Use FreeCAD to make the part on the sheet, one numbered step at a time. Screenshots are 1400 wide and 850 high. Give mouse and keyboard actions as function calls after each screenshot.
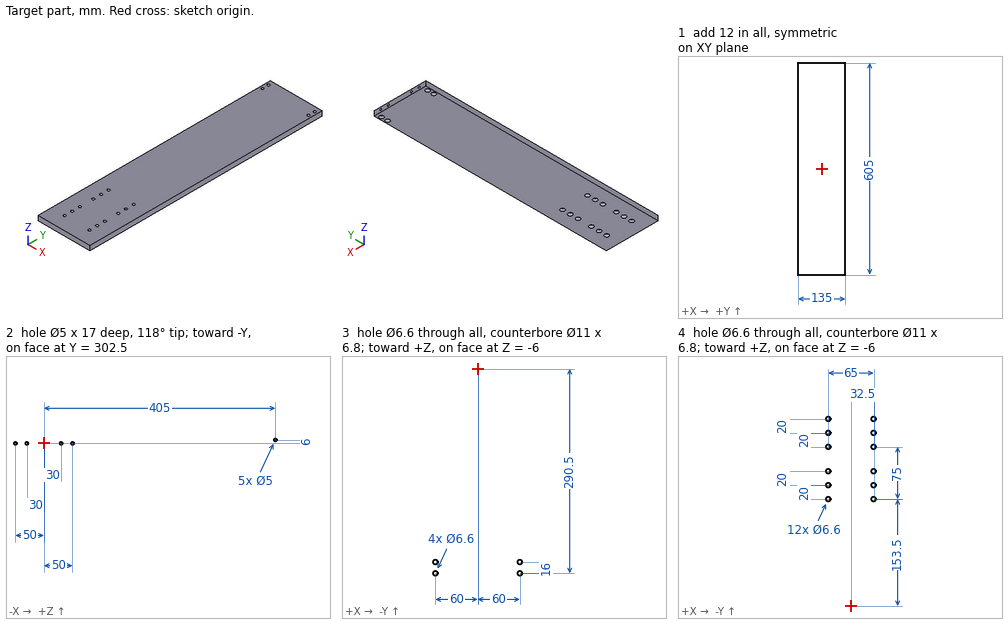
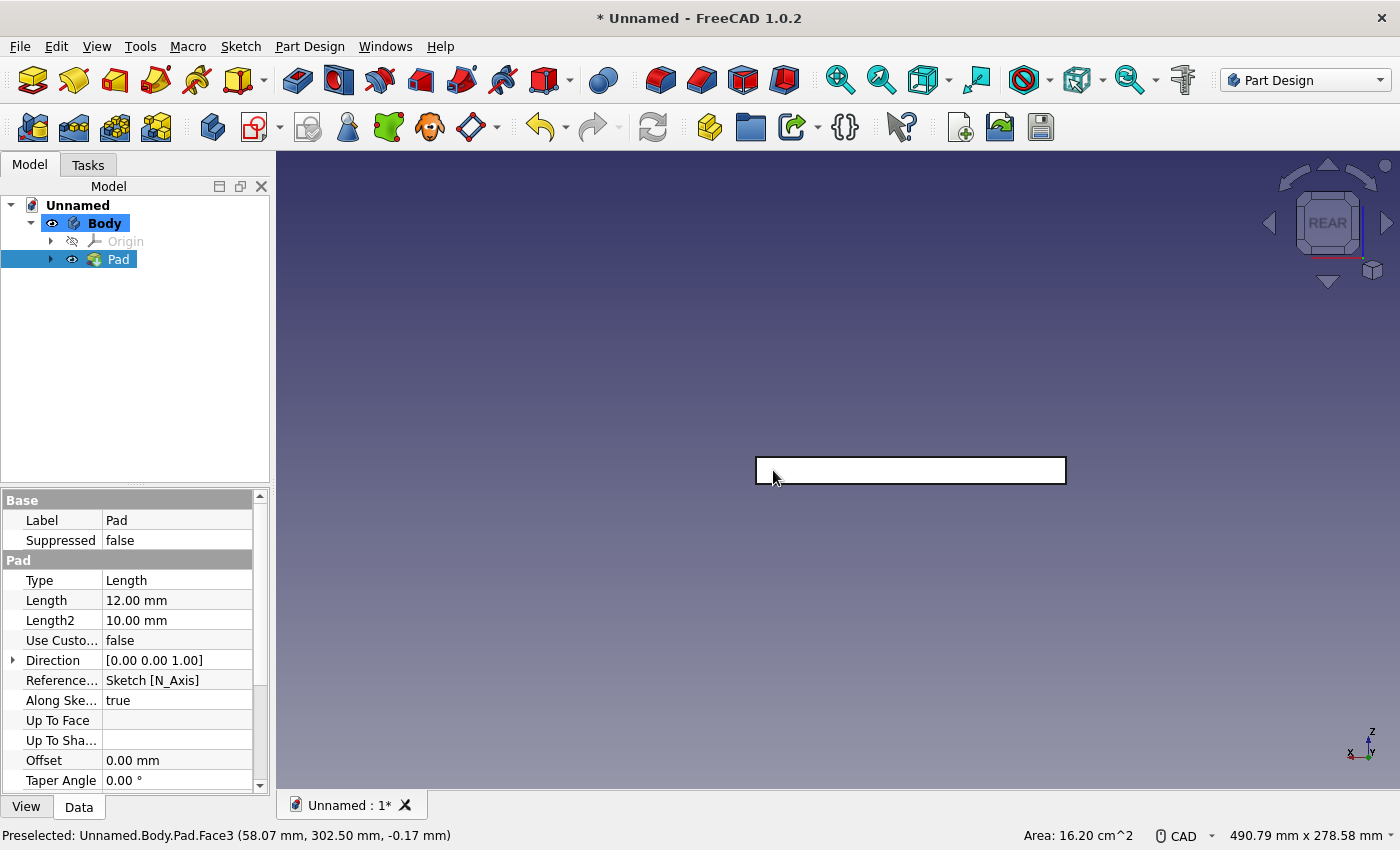
click(254, 128)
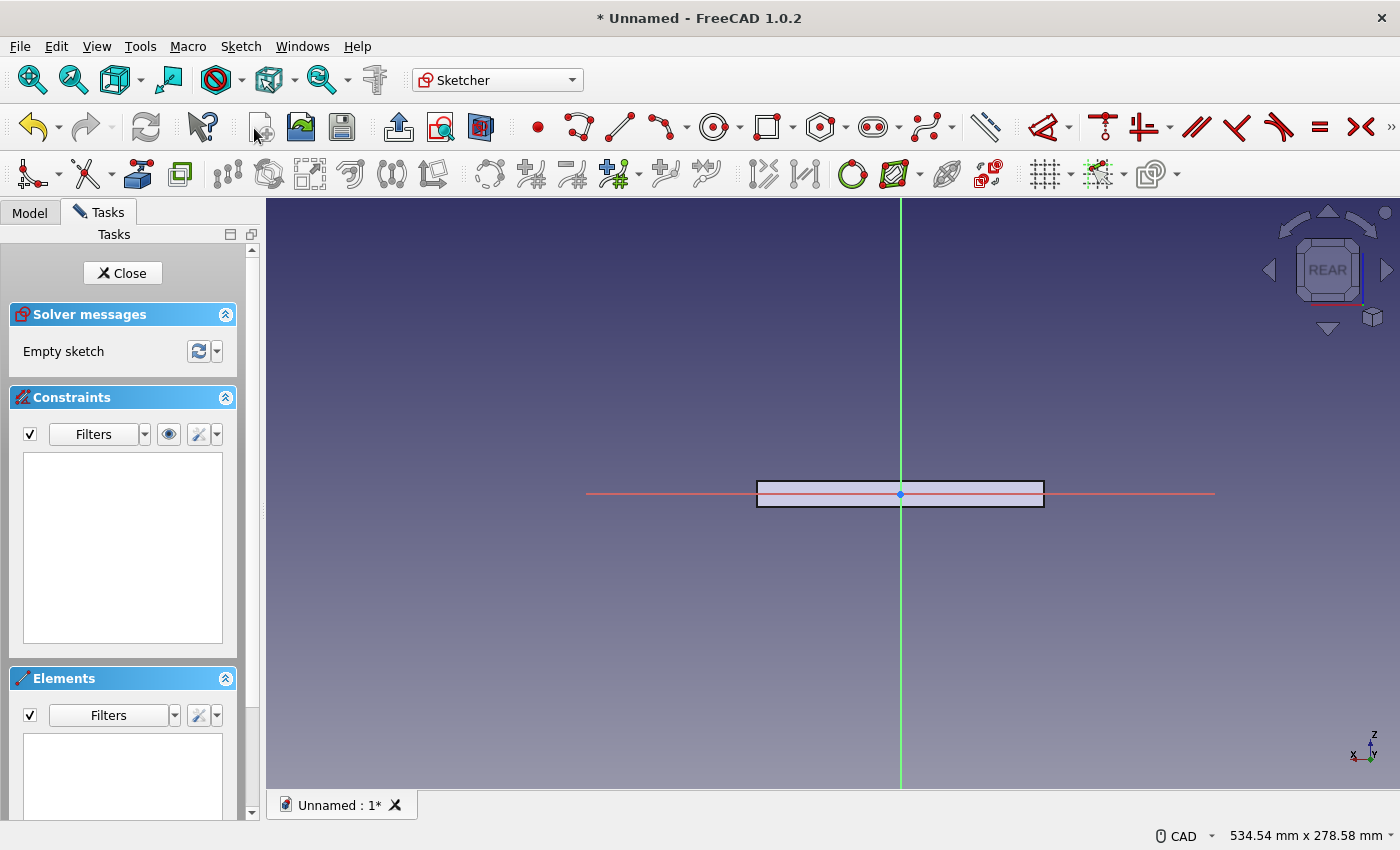
scroll(294, 501, down, 3)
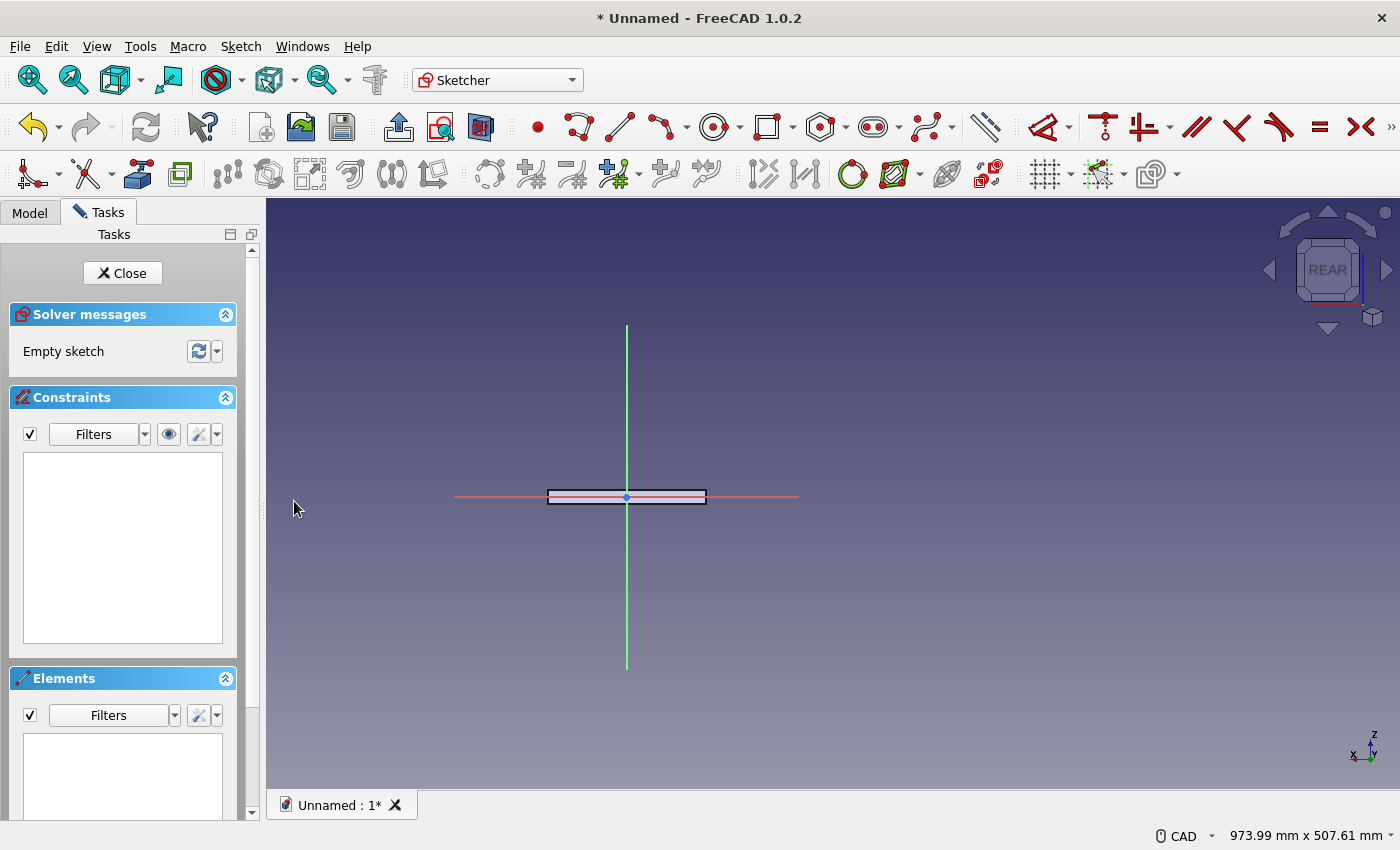
key(g)
key(c)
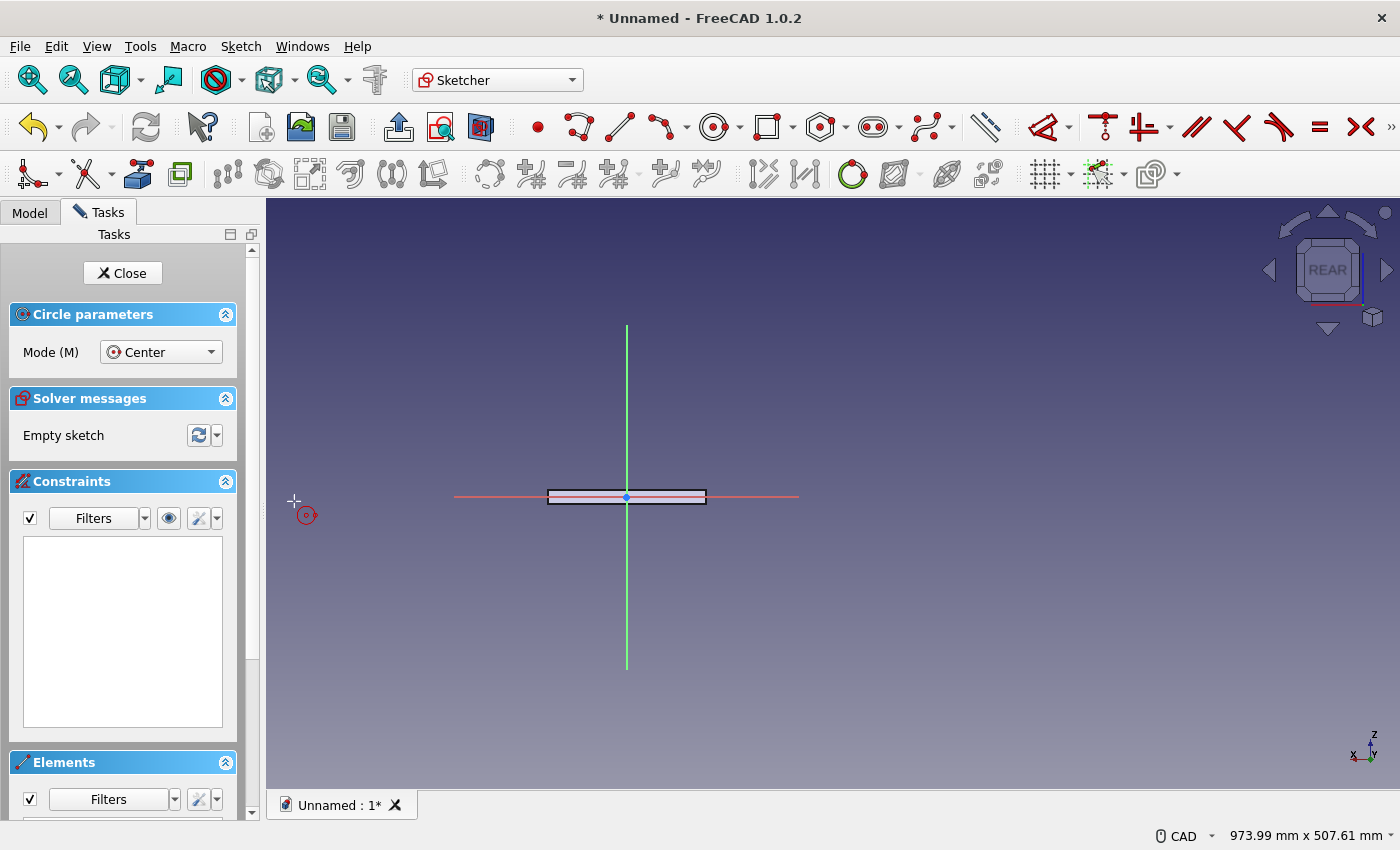
scroll(569, 497, up, 11)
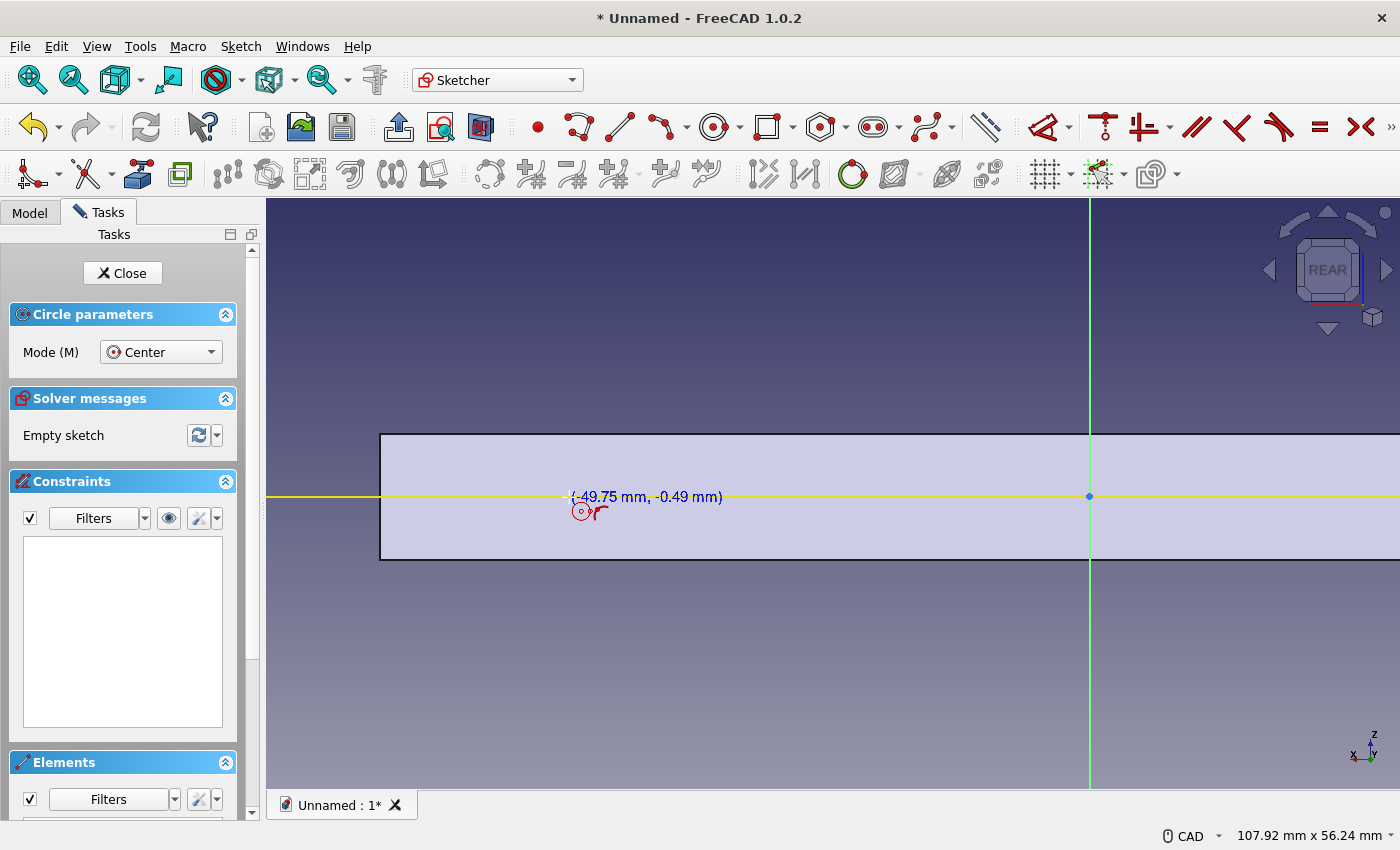
scroll(422, 498, down, 10)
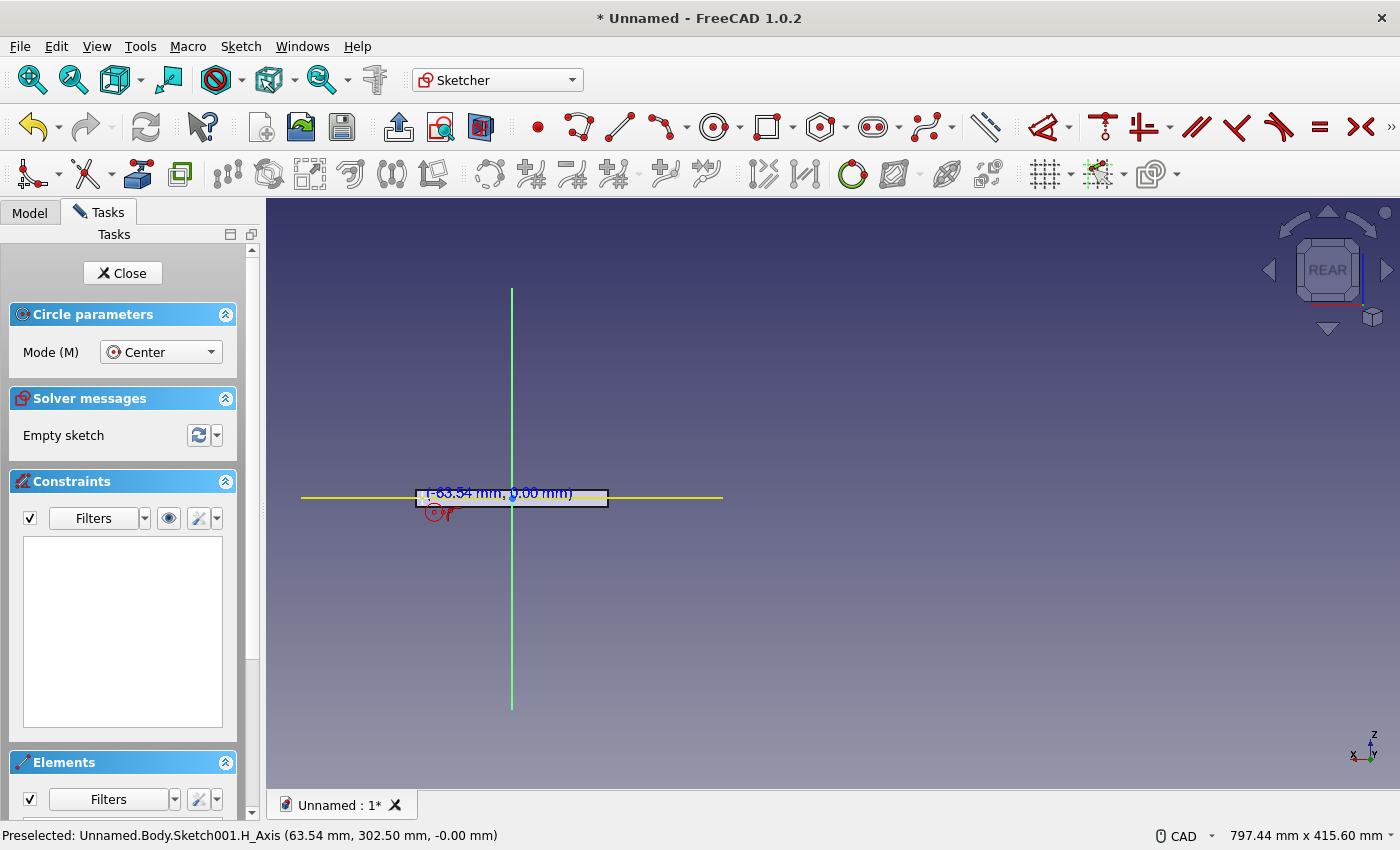
click(441, 498)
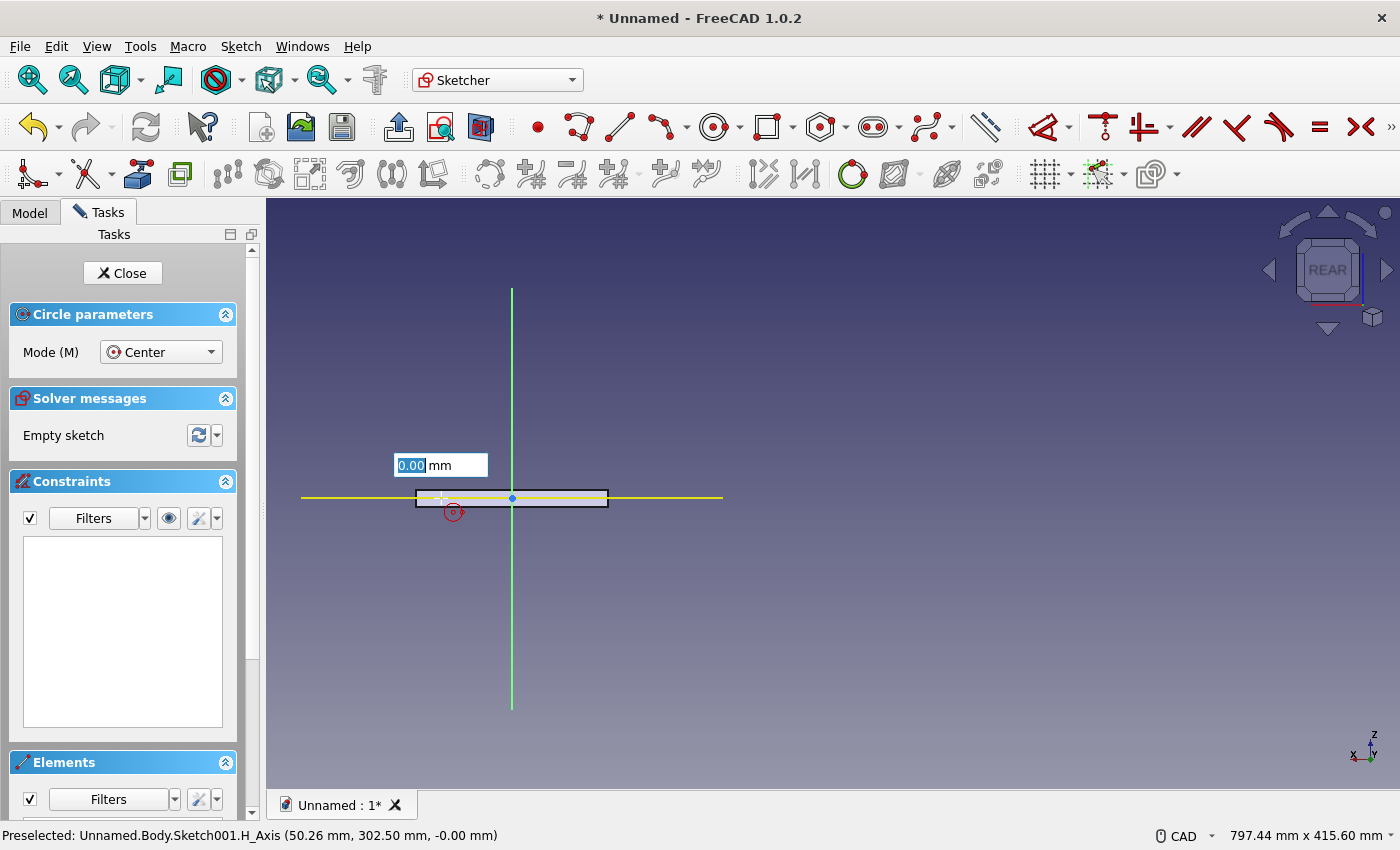
scroll(440, 502, up, 8)
move(440, 498)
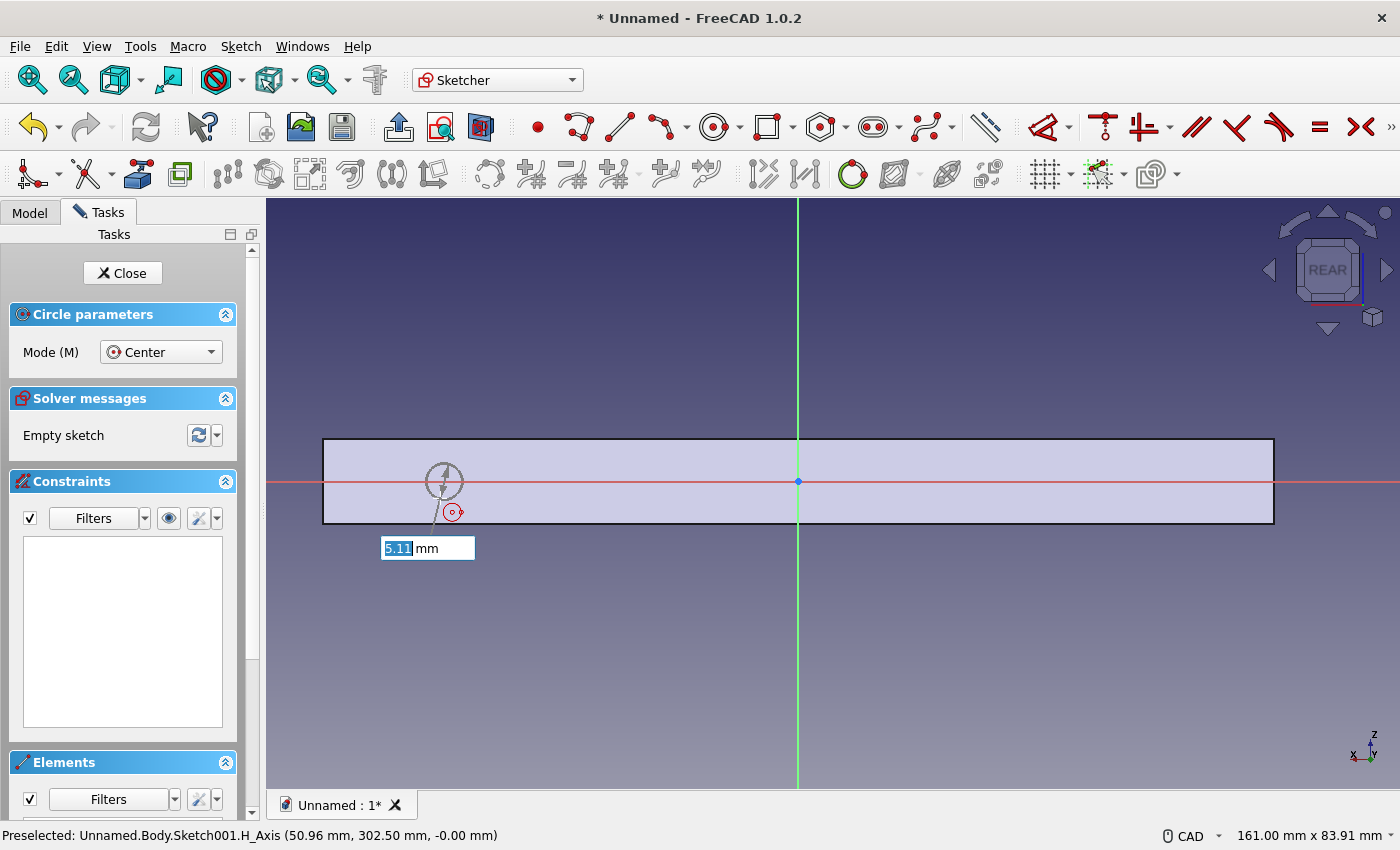
text(5)
key(Return)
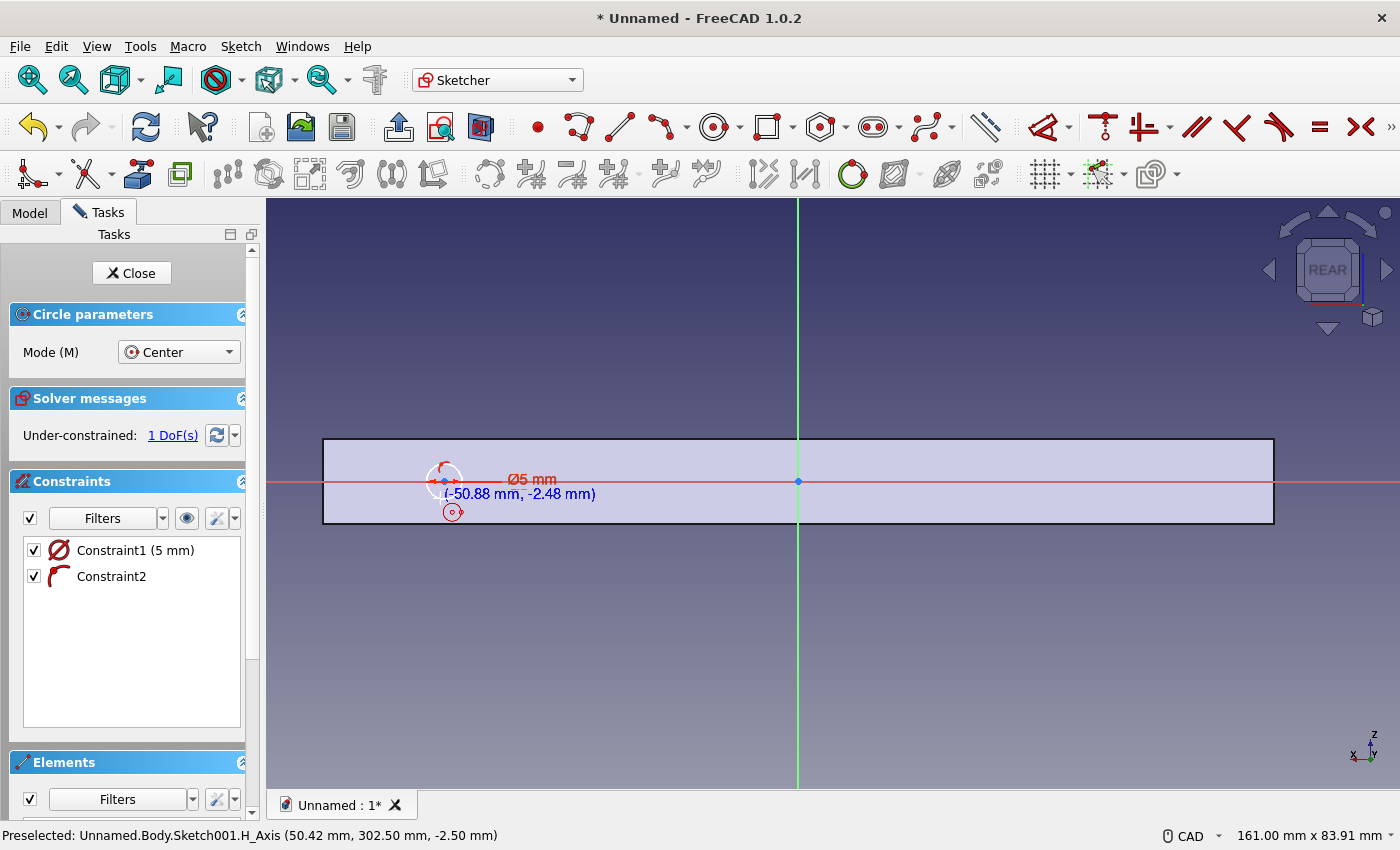
scroll(1010, 482, up, 2)